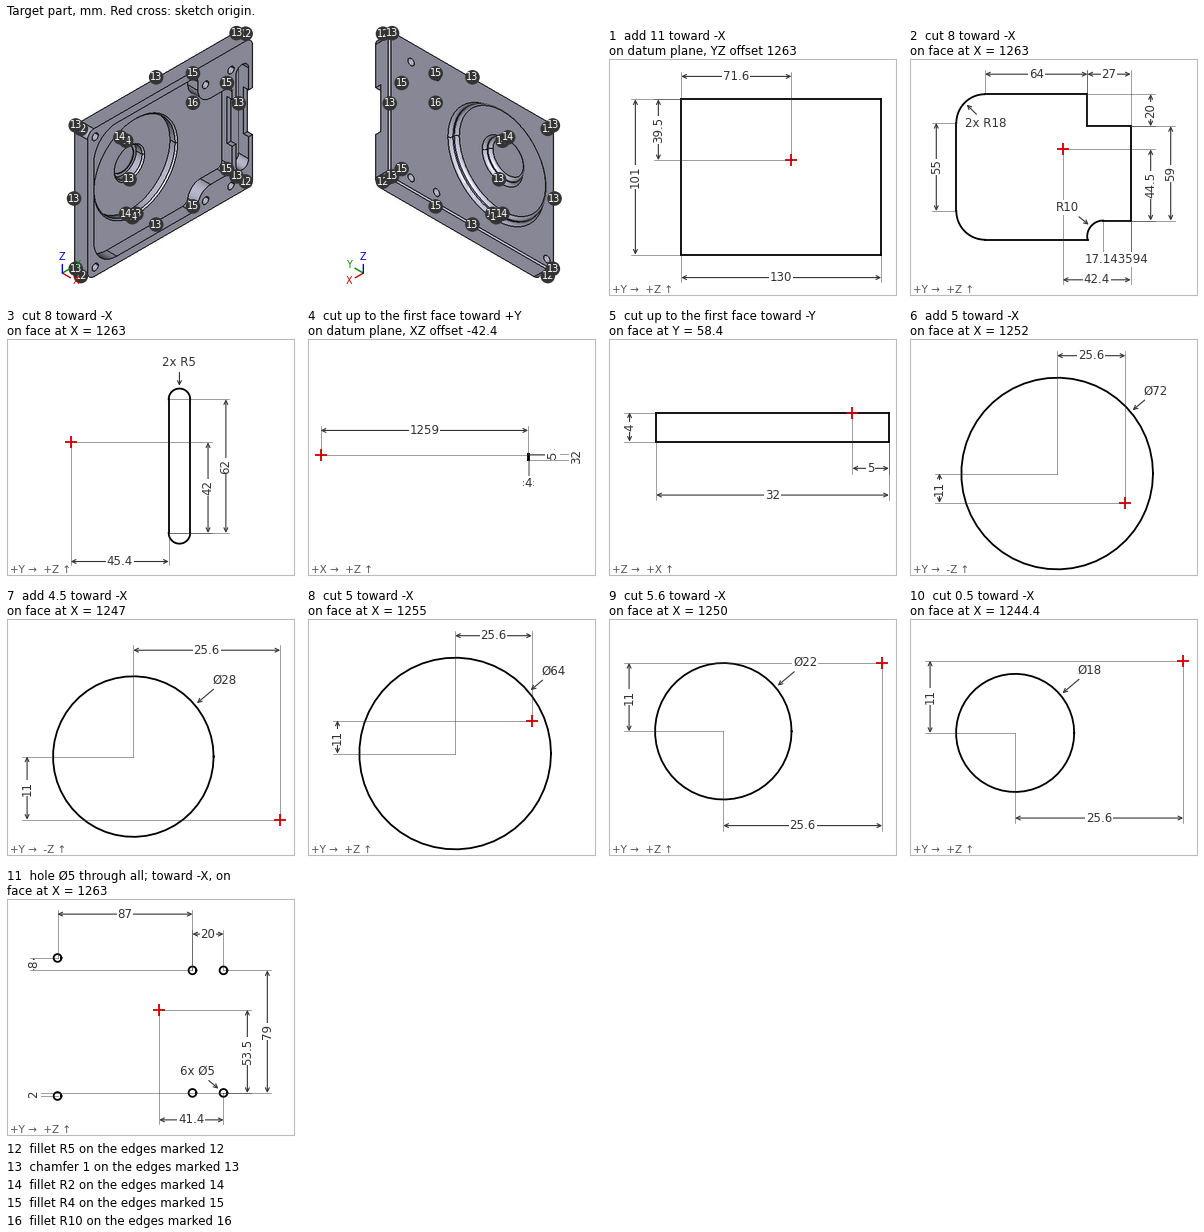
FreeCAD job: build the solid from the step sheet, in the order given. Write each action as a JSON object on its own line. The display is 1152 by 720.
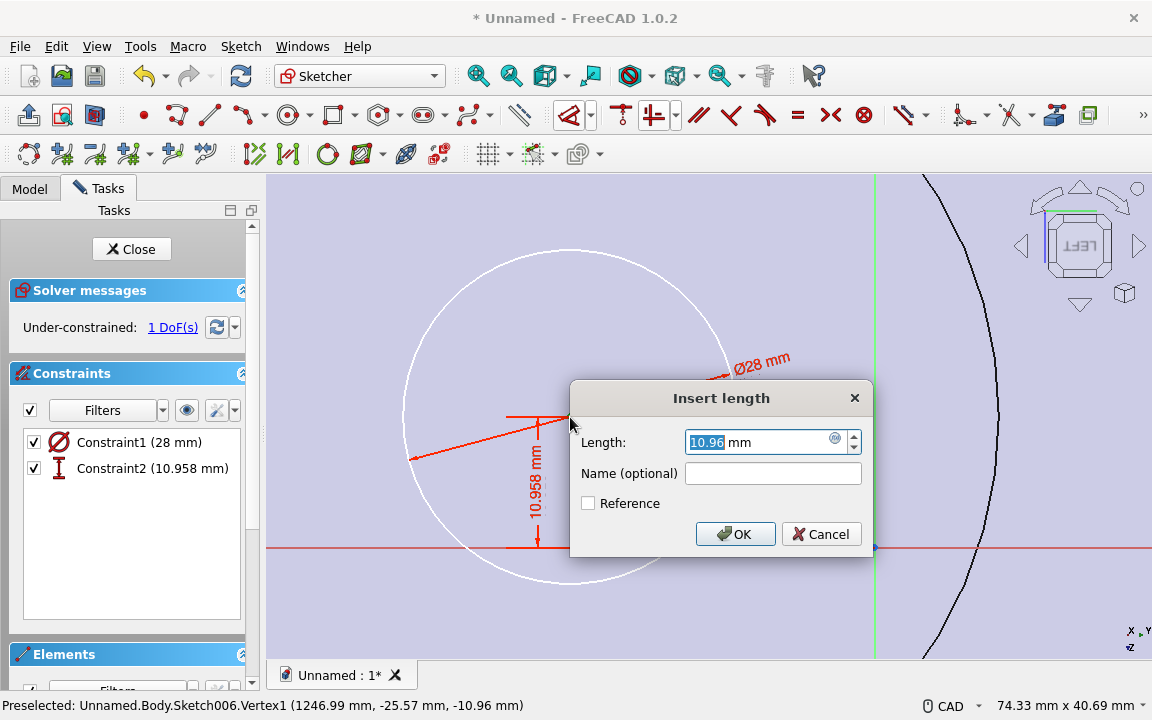
{"action": "type", "text": "11"}
{"action": "key", "text": "Return"}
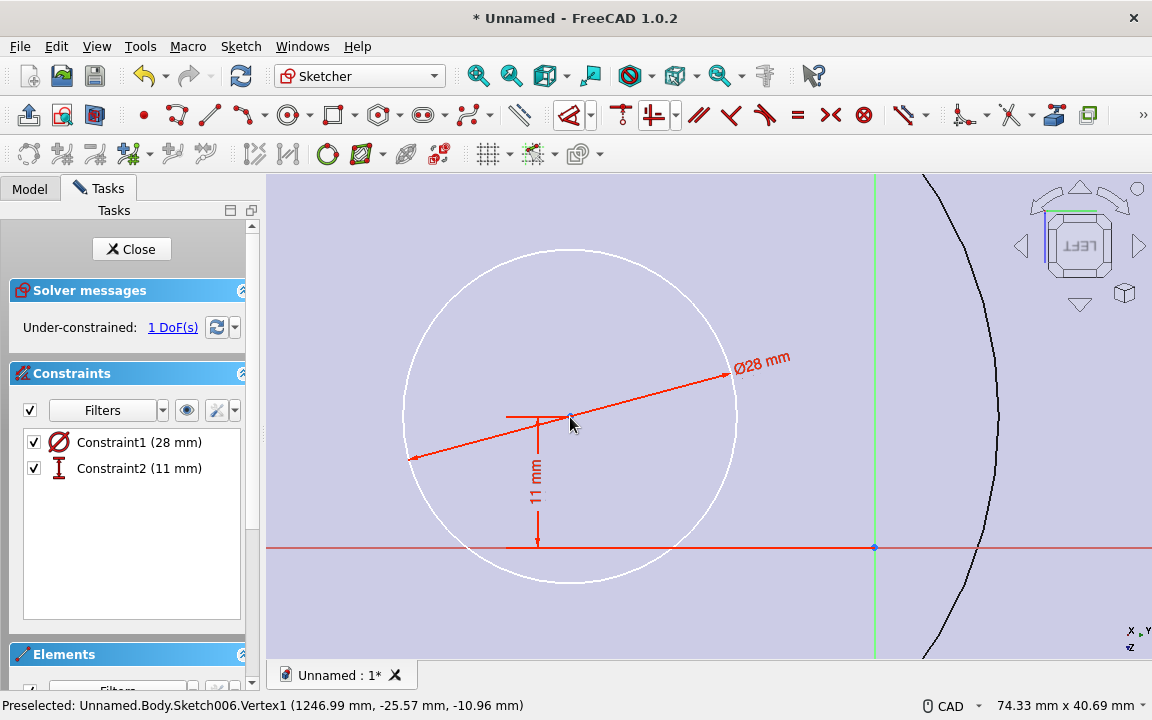
{"action": "left_click", "coordinate": [570, 416]}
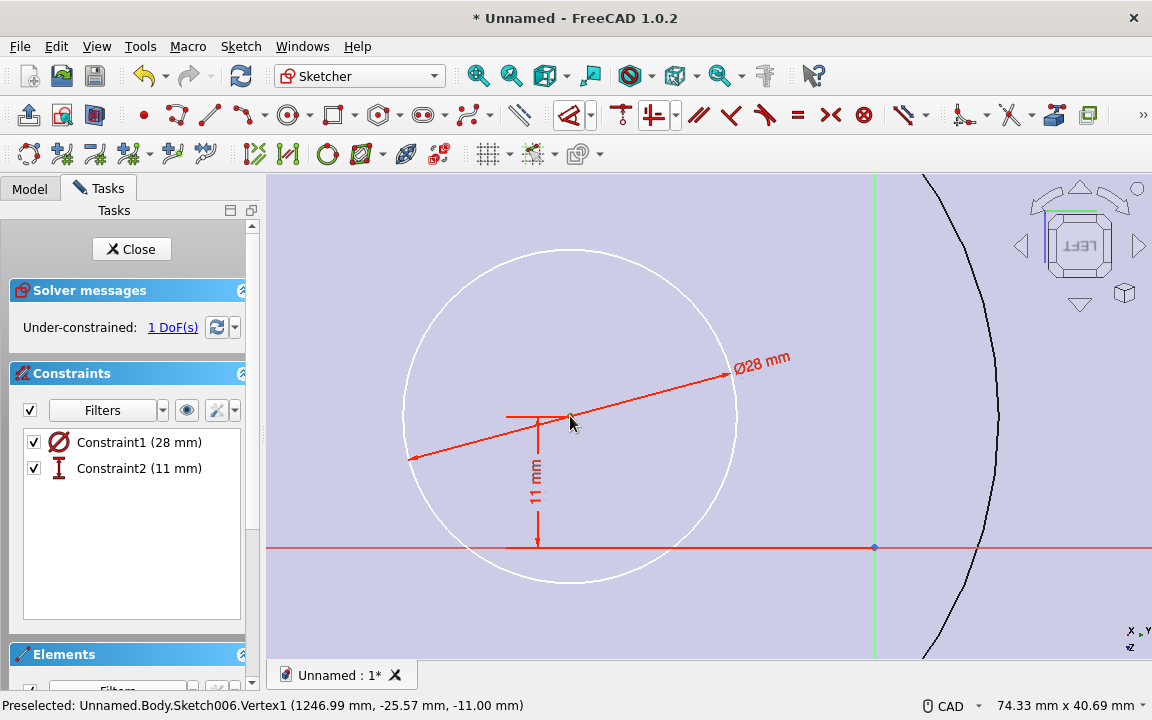
{"action": "key", "text": "l"}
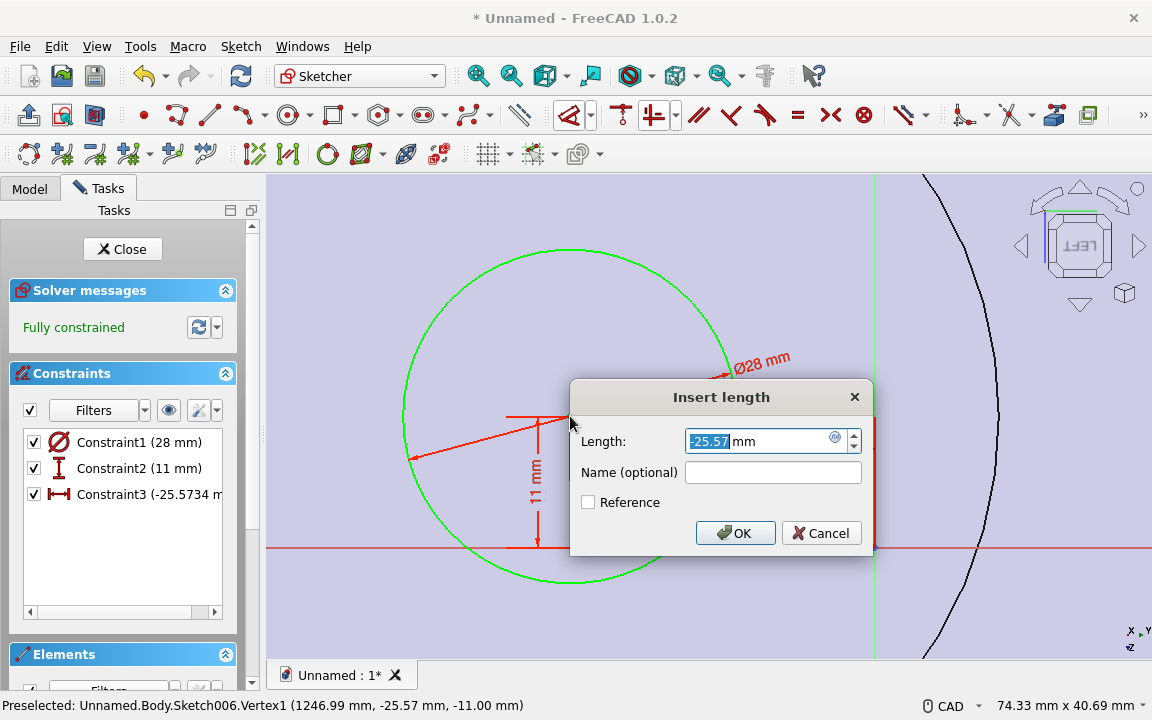
{"action": "type", "text": "-25.6"}
{"action": "key", "text": "Return"}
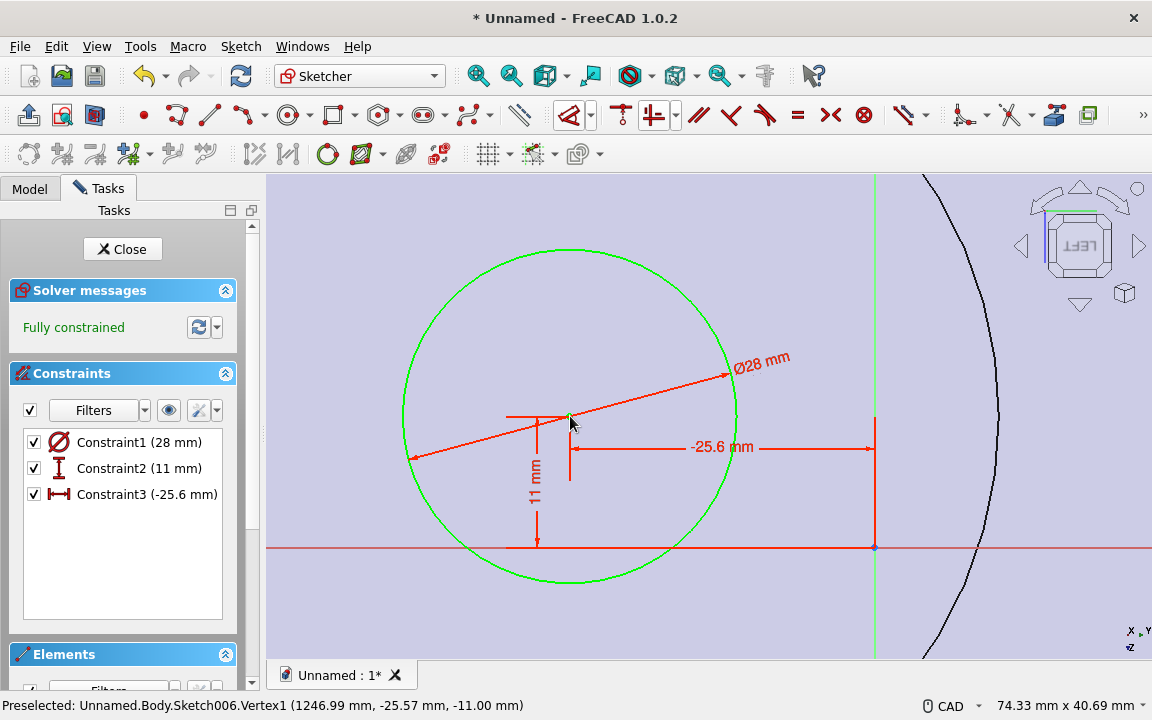
{"action": "left_click", "coordinate": [123, 249]}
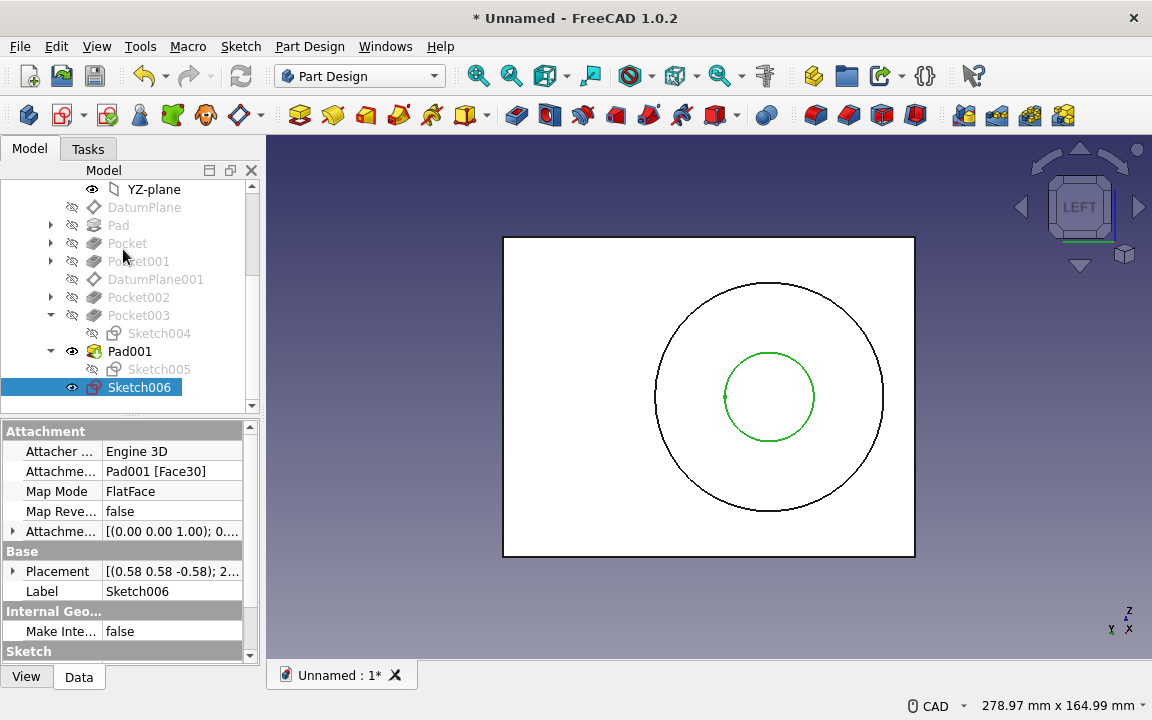
{"action": "left_click", "coordinate": [300, 116]}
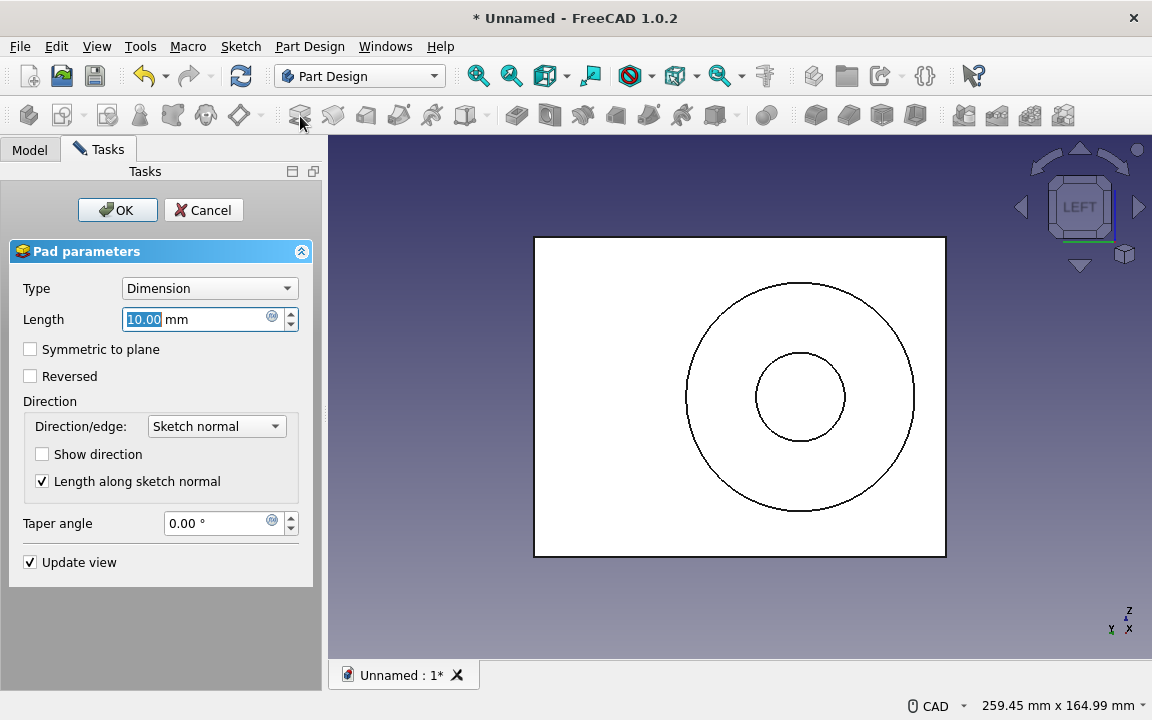
{"action": "type", "text": "4.5"}
{"action": "key", "text": "Tab"}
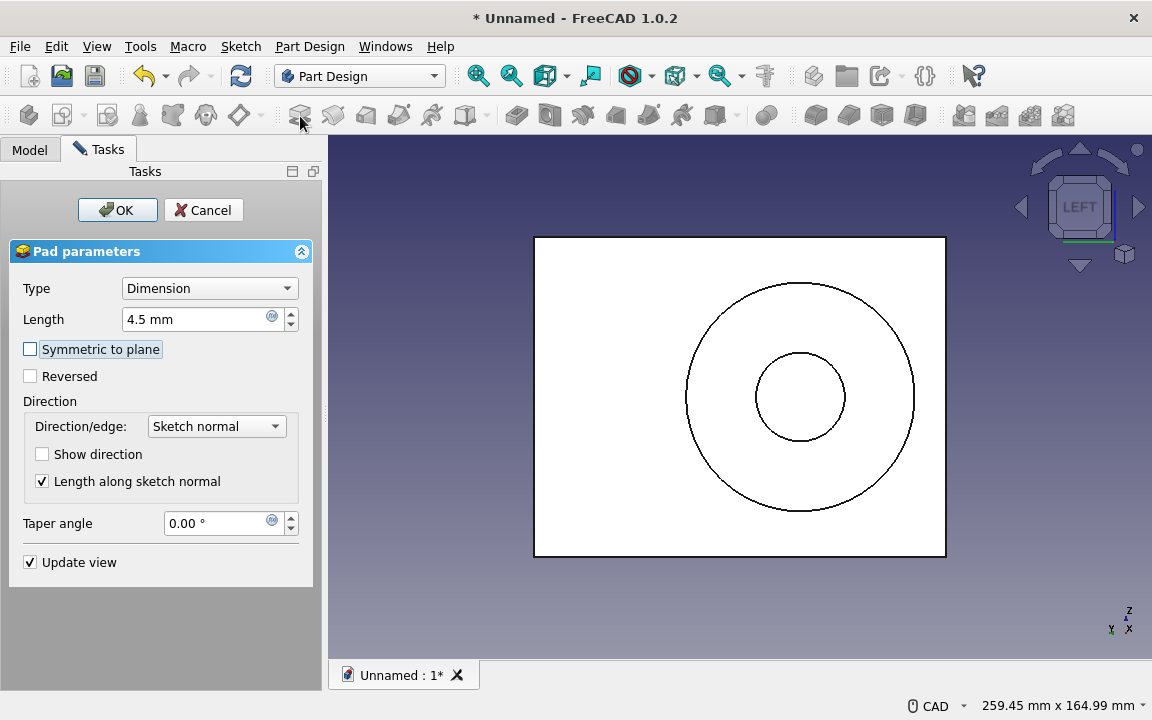
{"action": "left_click", "coordinate": [118, 210]}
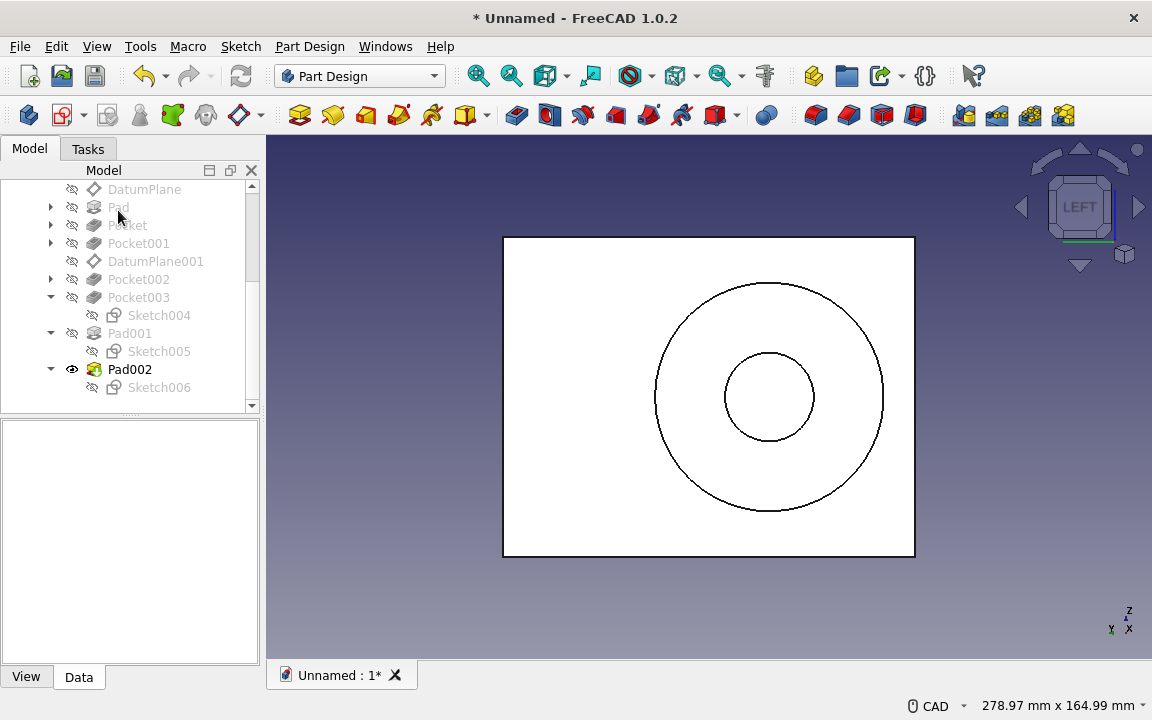
{"action": "key", "text": "0"}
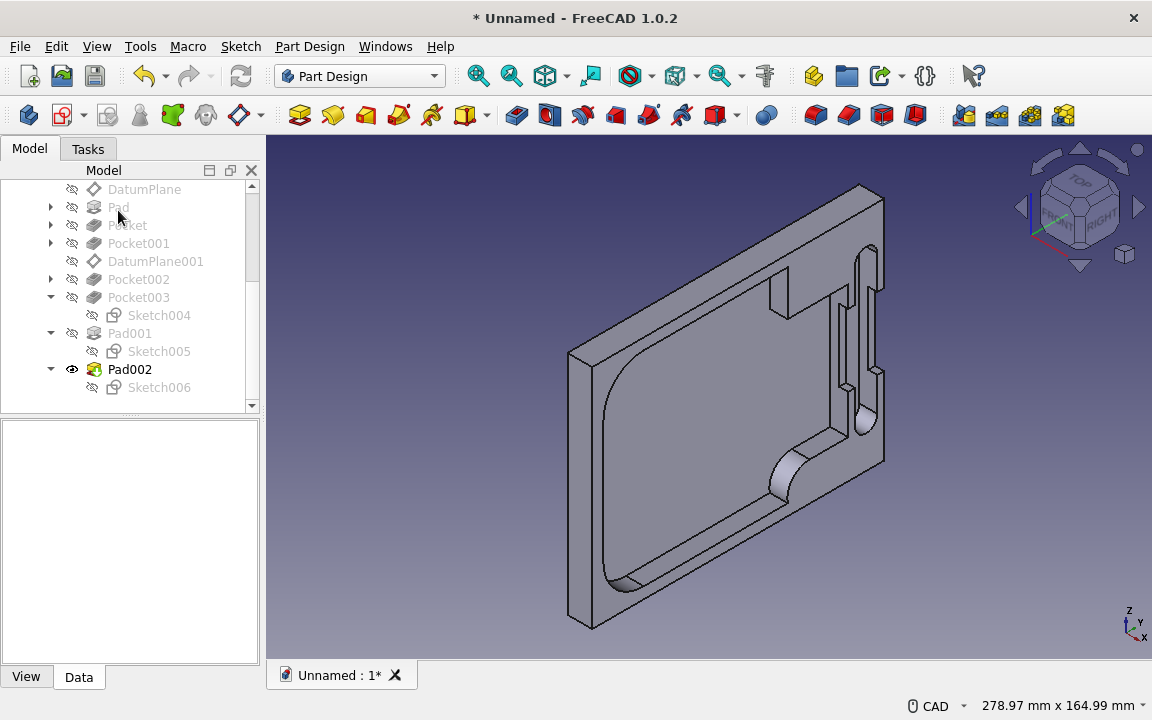
{"action": "left_click", "coordinate": [673, 430]}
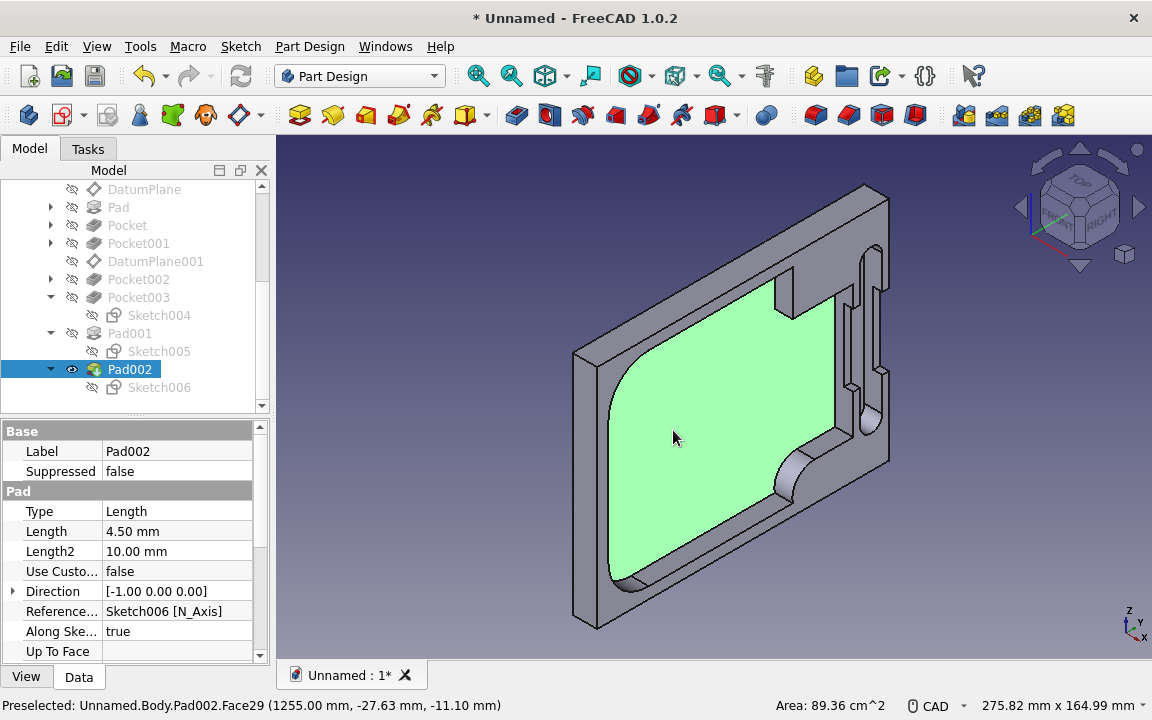
{"action": "left_click", "coordinate": [62, 116]}